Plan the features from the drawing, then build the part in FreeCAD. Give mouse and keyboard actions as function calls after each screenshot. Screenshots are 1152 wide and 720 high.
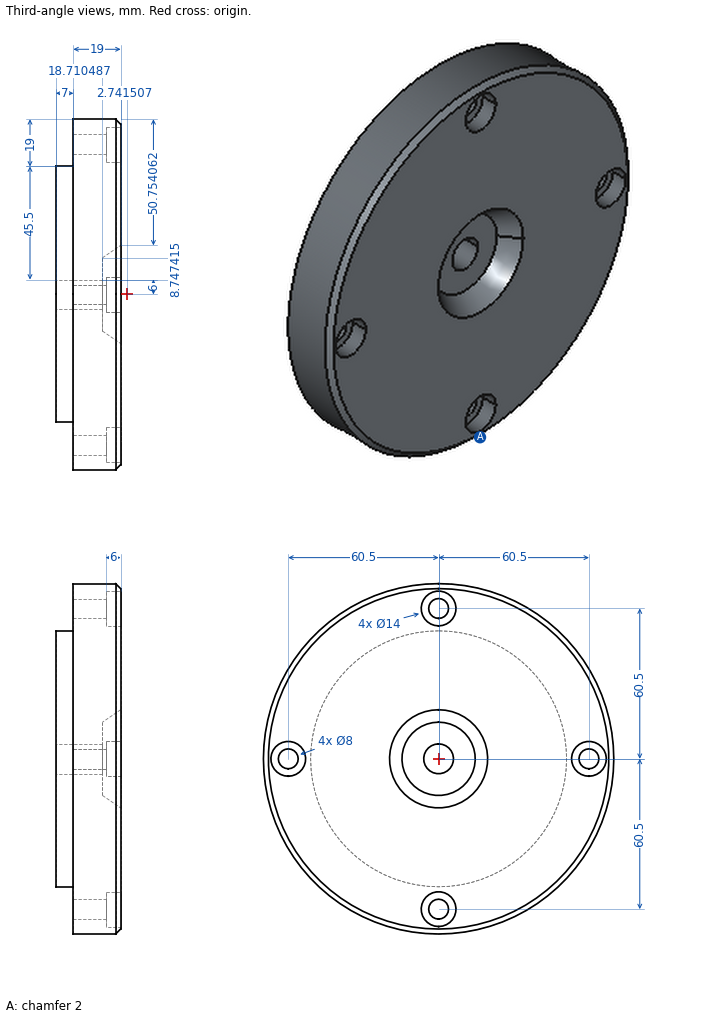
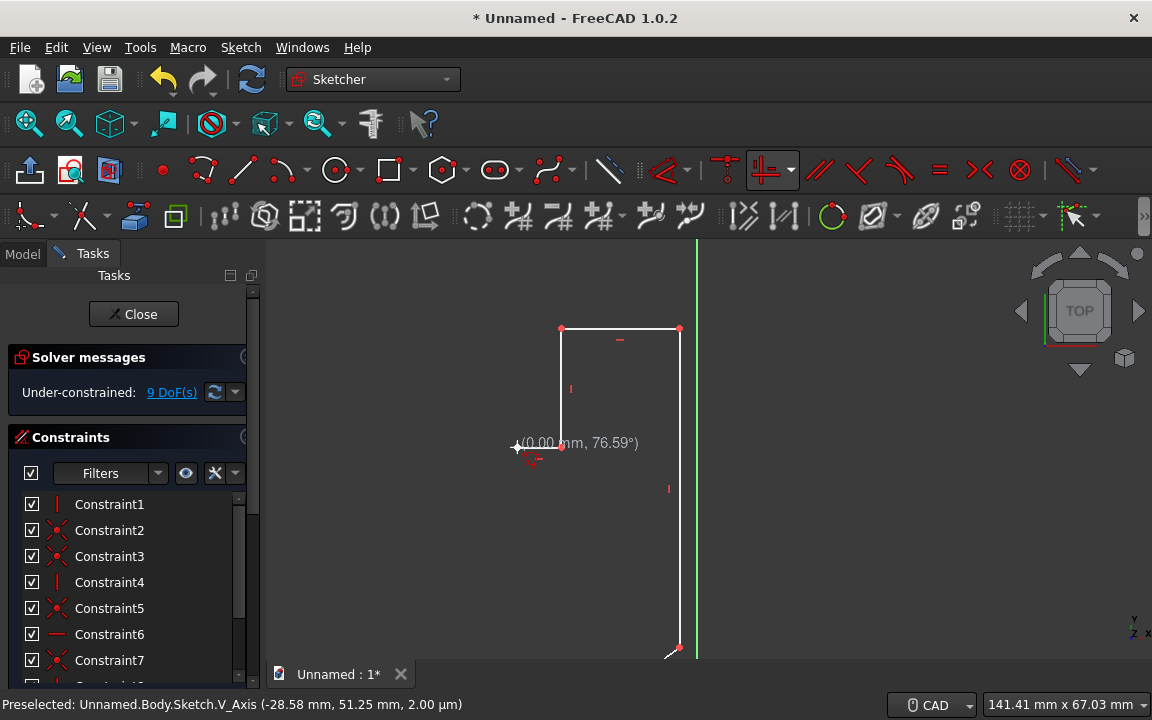
scroll(681, 327, down, 3)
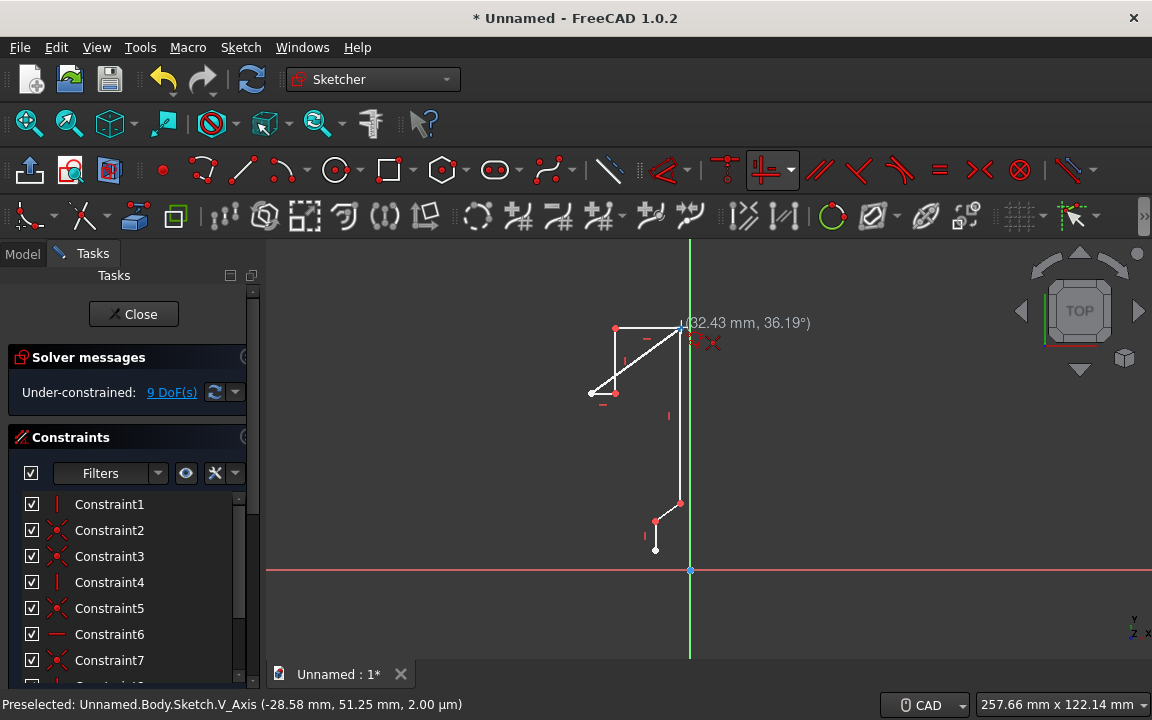
click(591, 550)
click(656, 550)
key(Escape)
key(Escape)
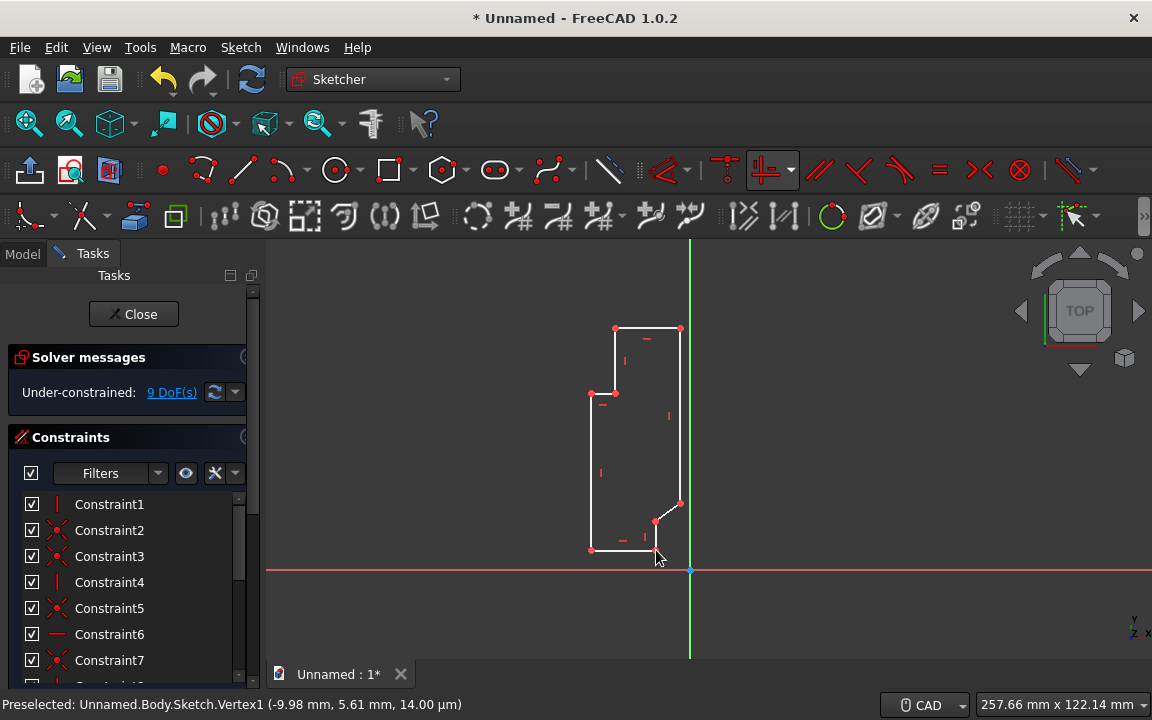
key(d)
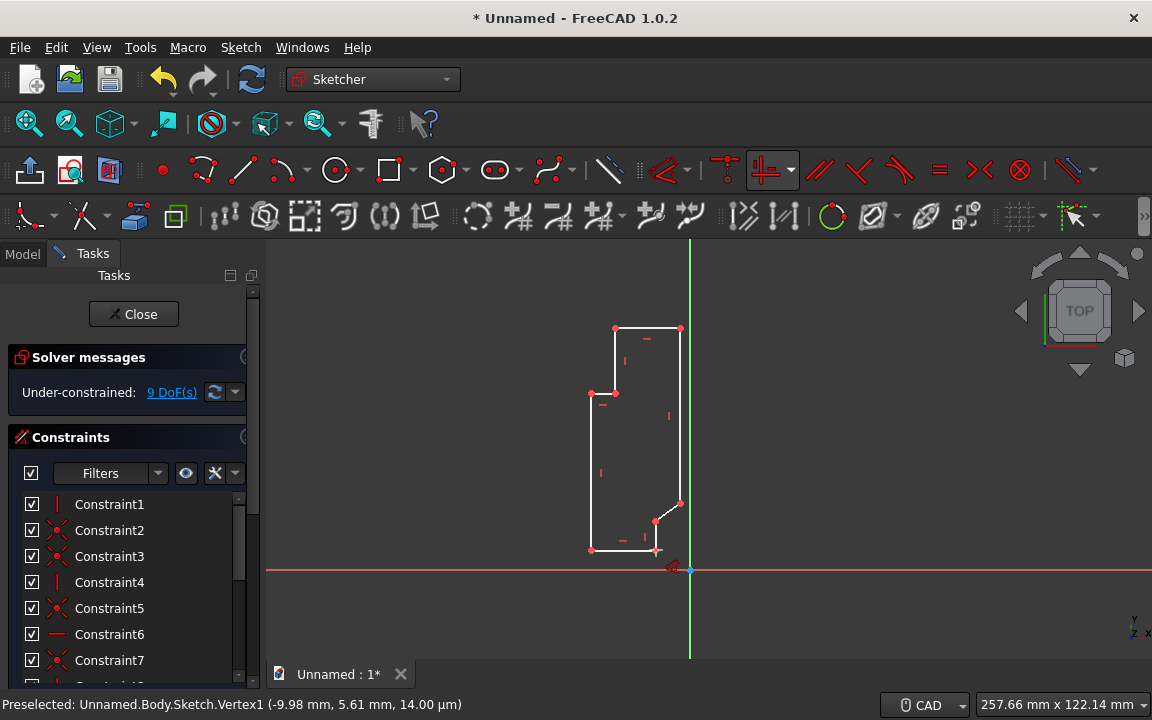
scroll(606, 394, up, 3)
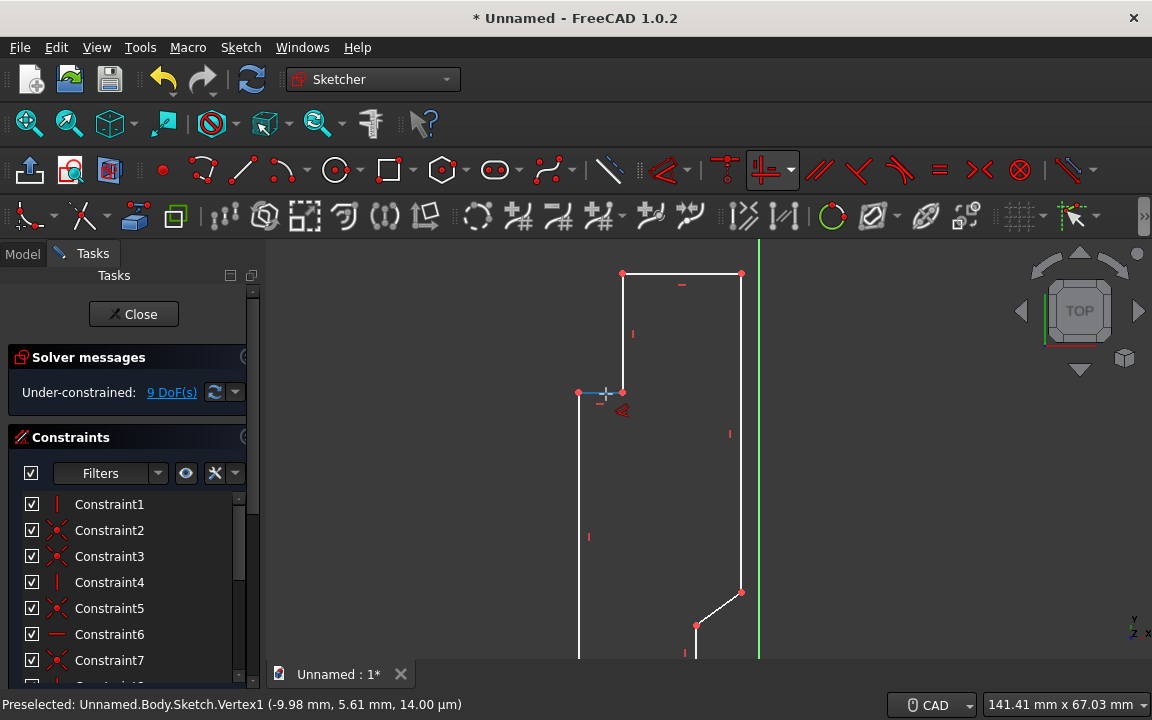
click(605, 393)
click(601, 359)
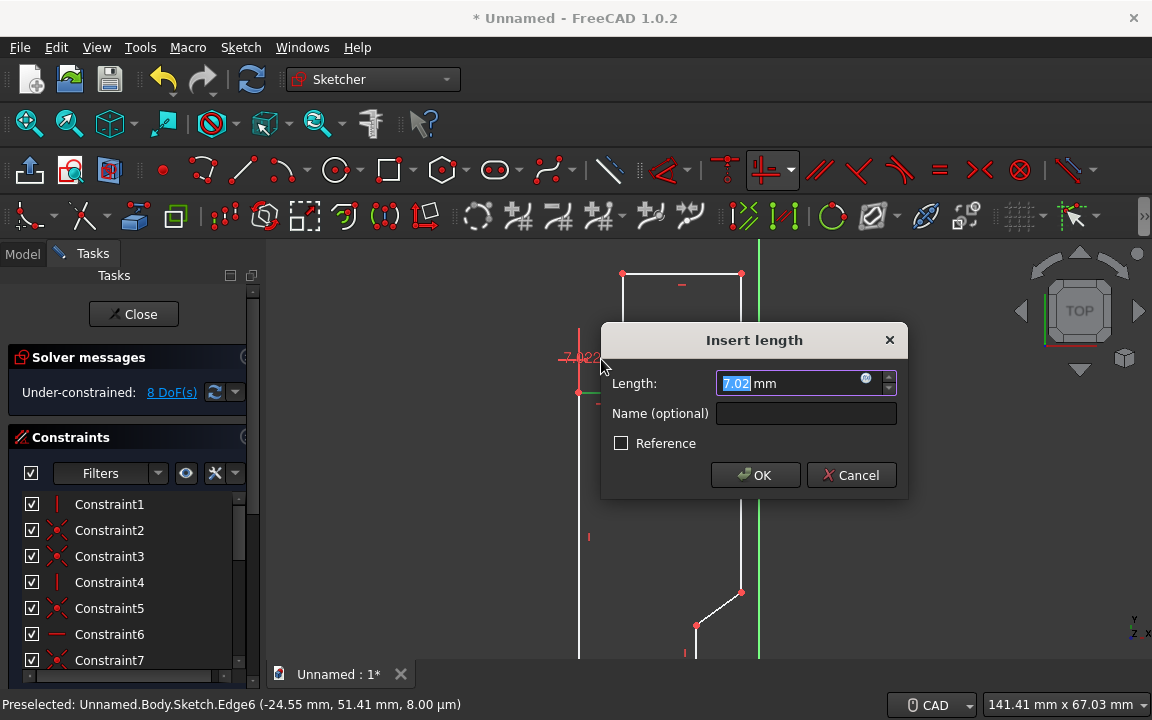
text(7)
key(Return)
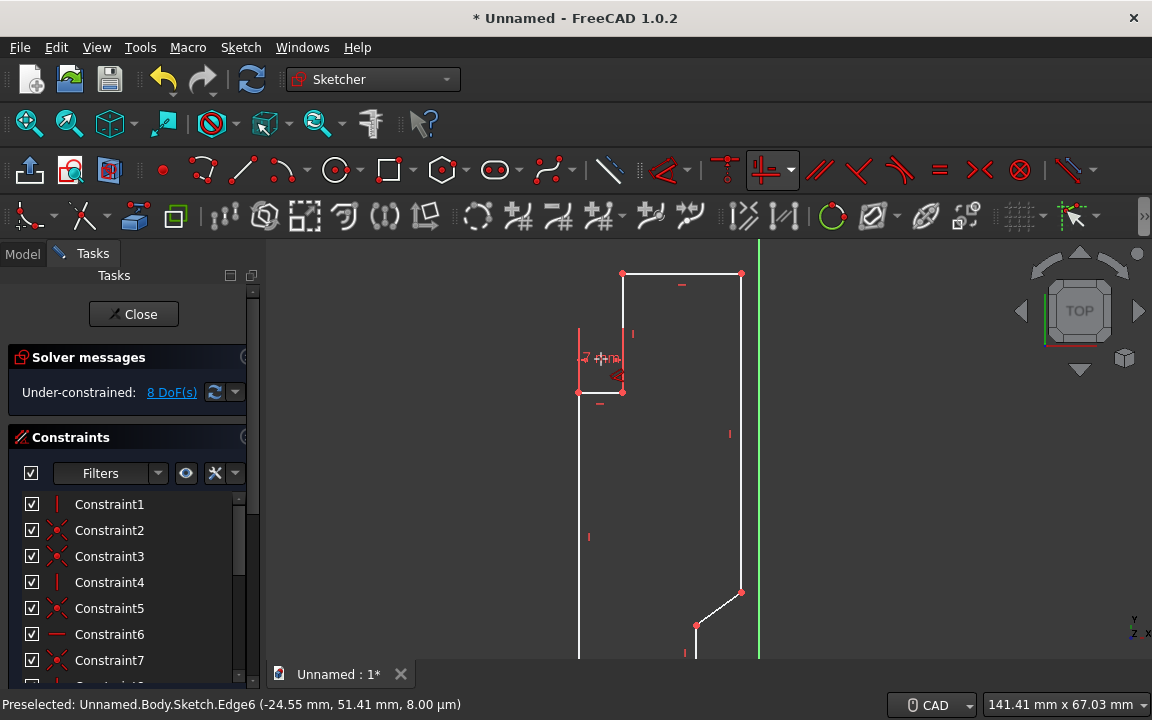
click(706, 274)
click(682, 308)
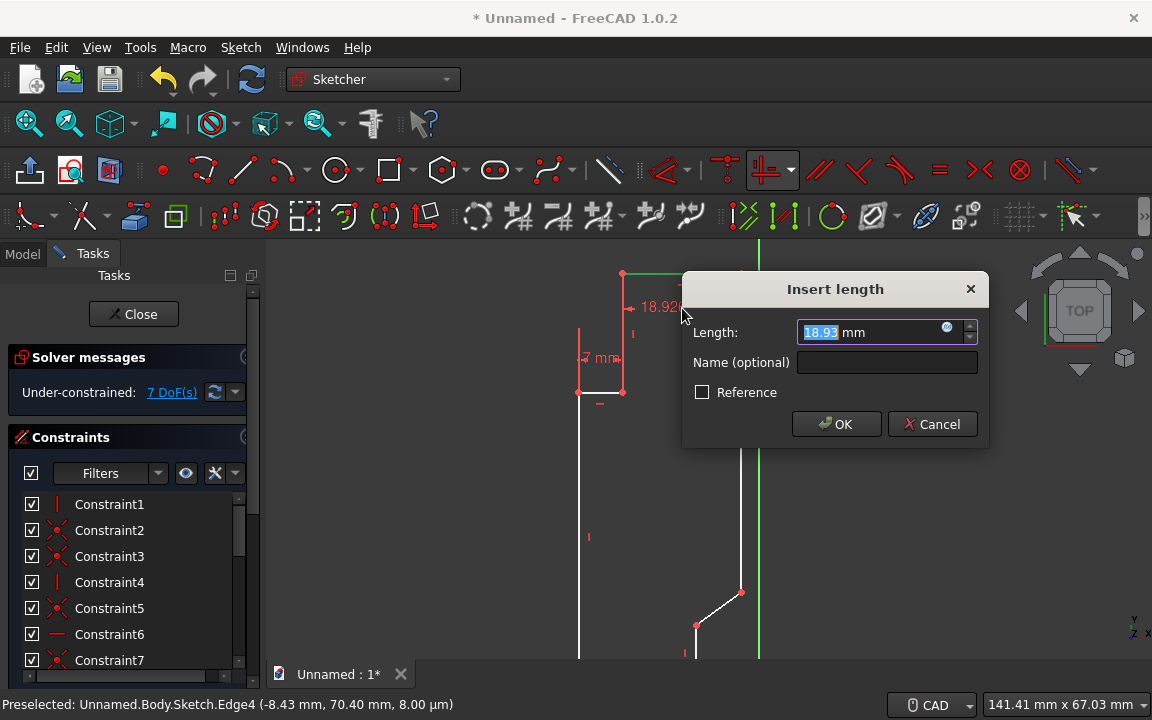
text(19)
key(Return)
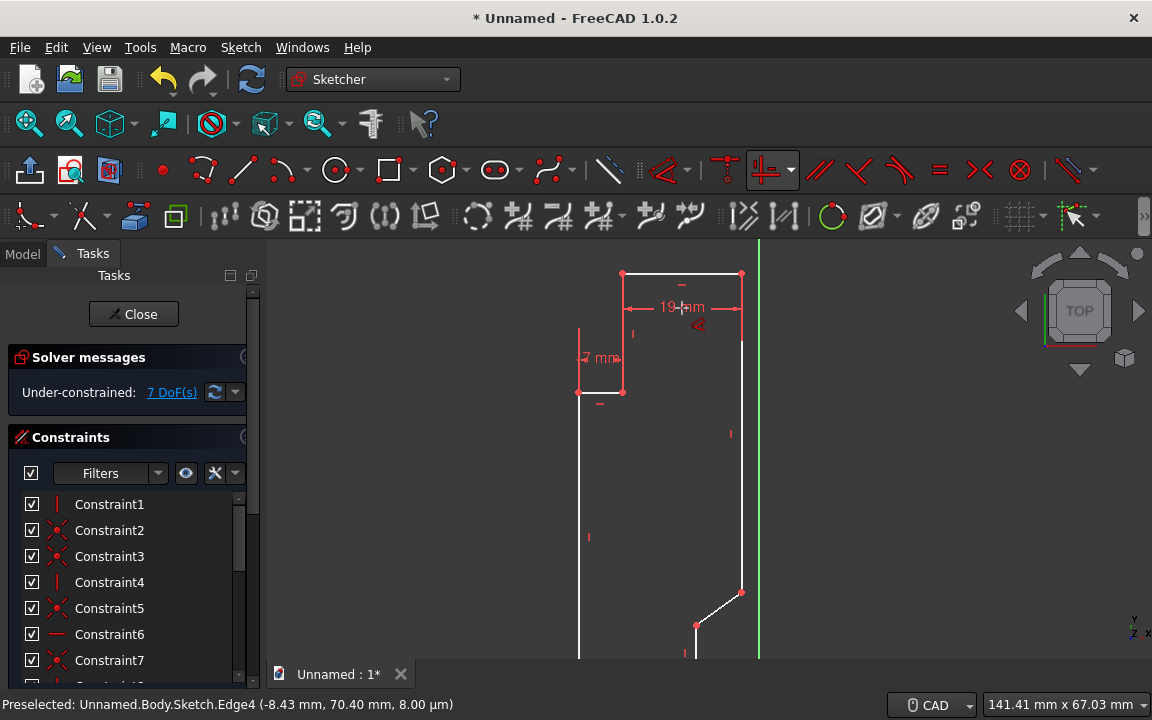
click(623, 309)
click(589, 333)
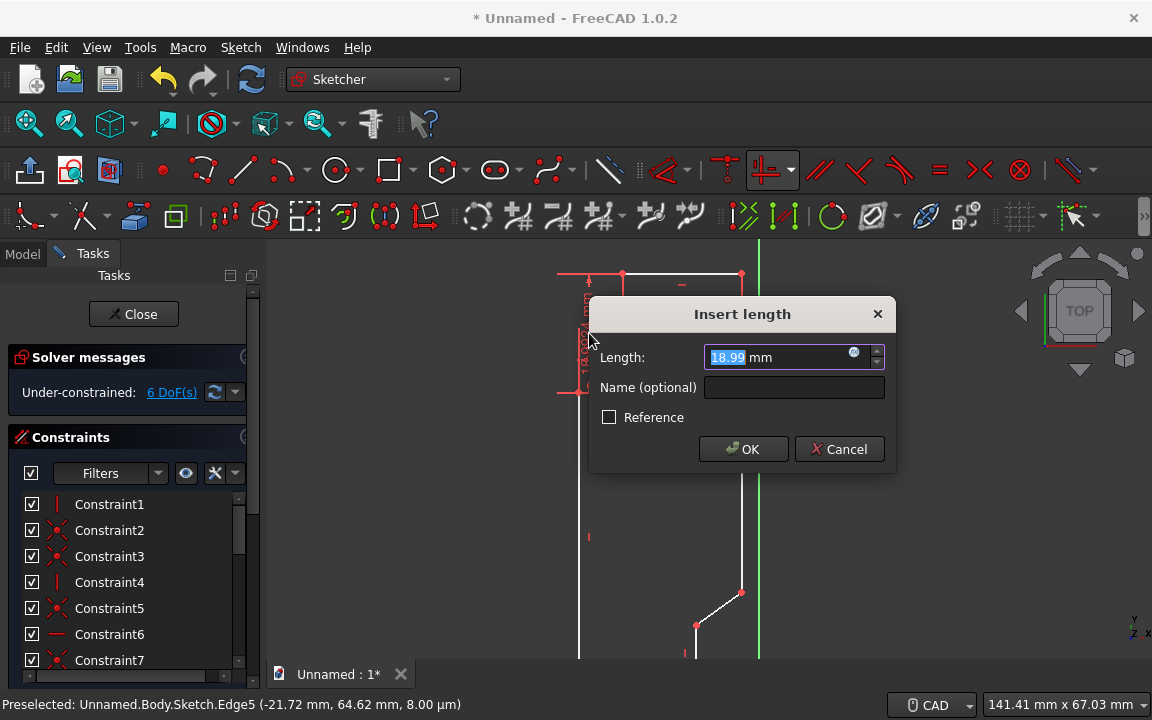
text(19)
key(Return)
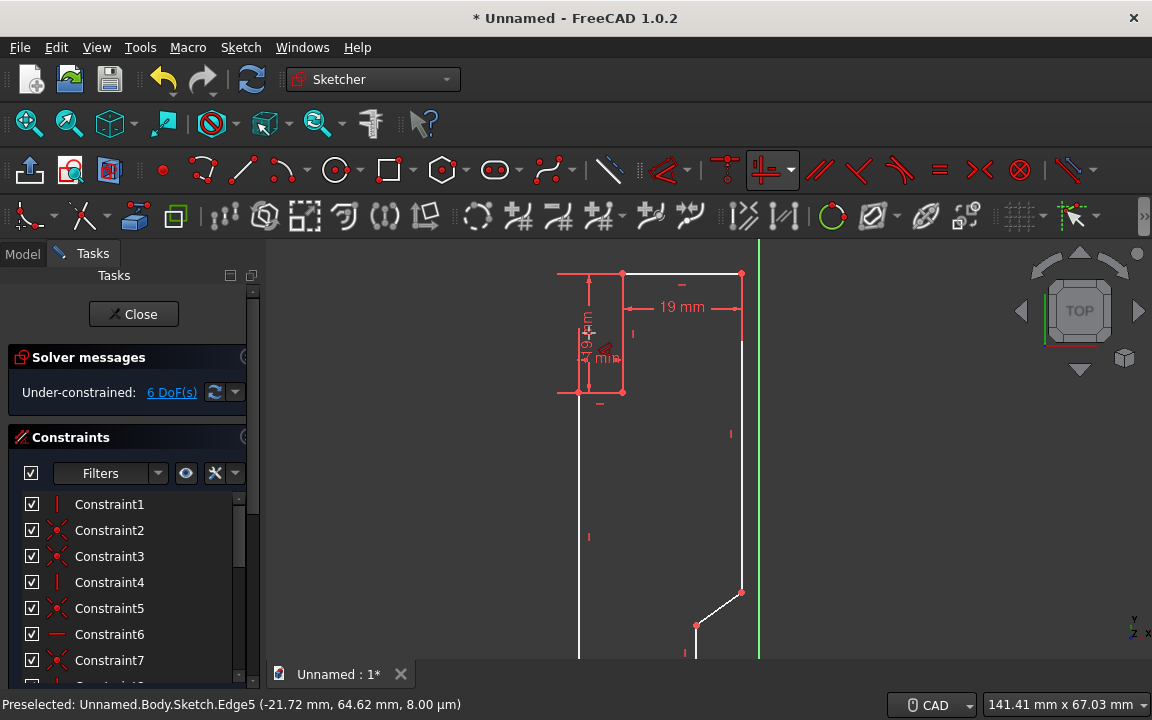
scroll(606, 394, down, 3)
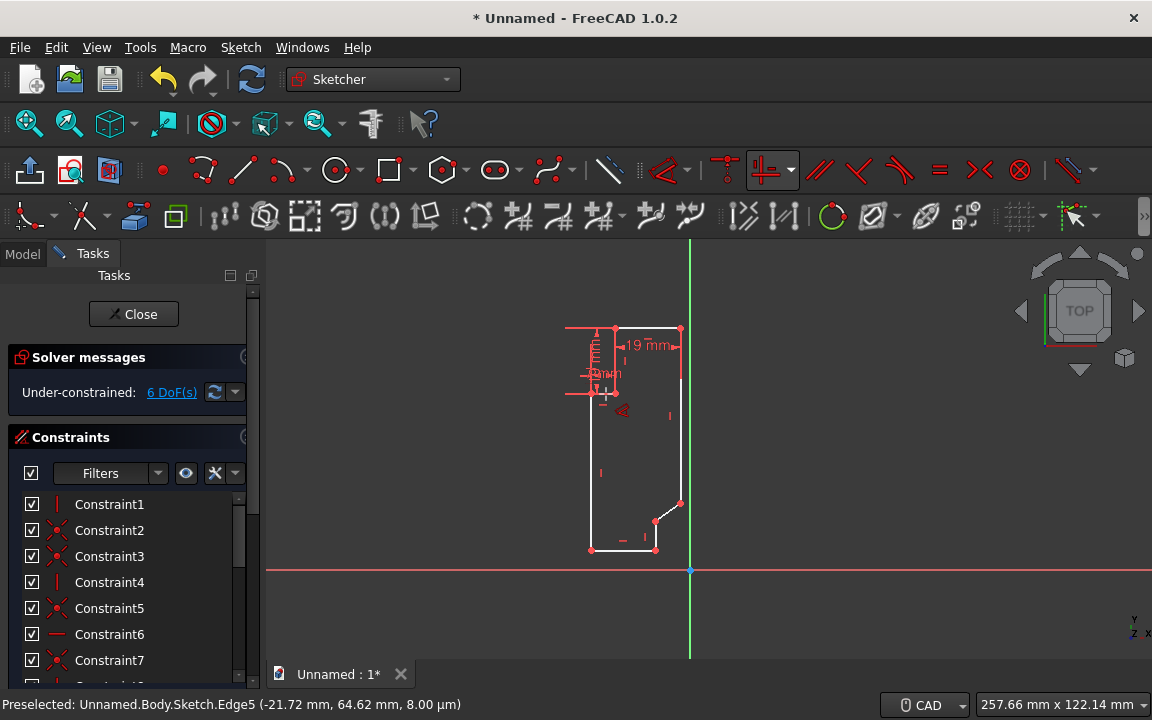
scroll(656, 551, up, 4)